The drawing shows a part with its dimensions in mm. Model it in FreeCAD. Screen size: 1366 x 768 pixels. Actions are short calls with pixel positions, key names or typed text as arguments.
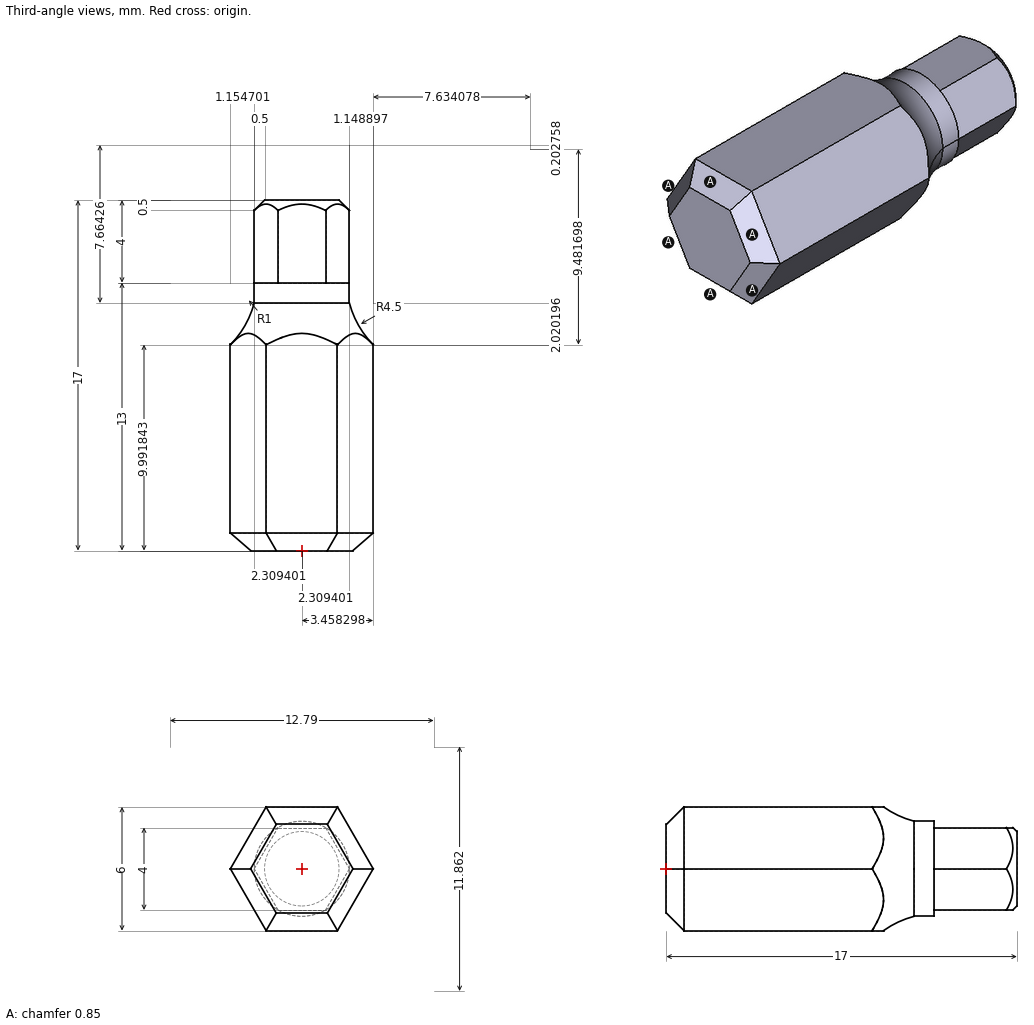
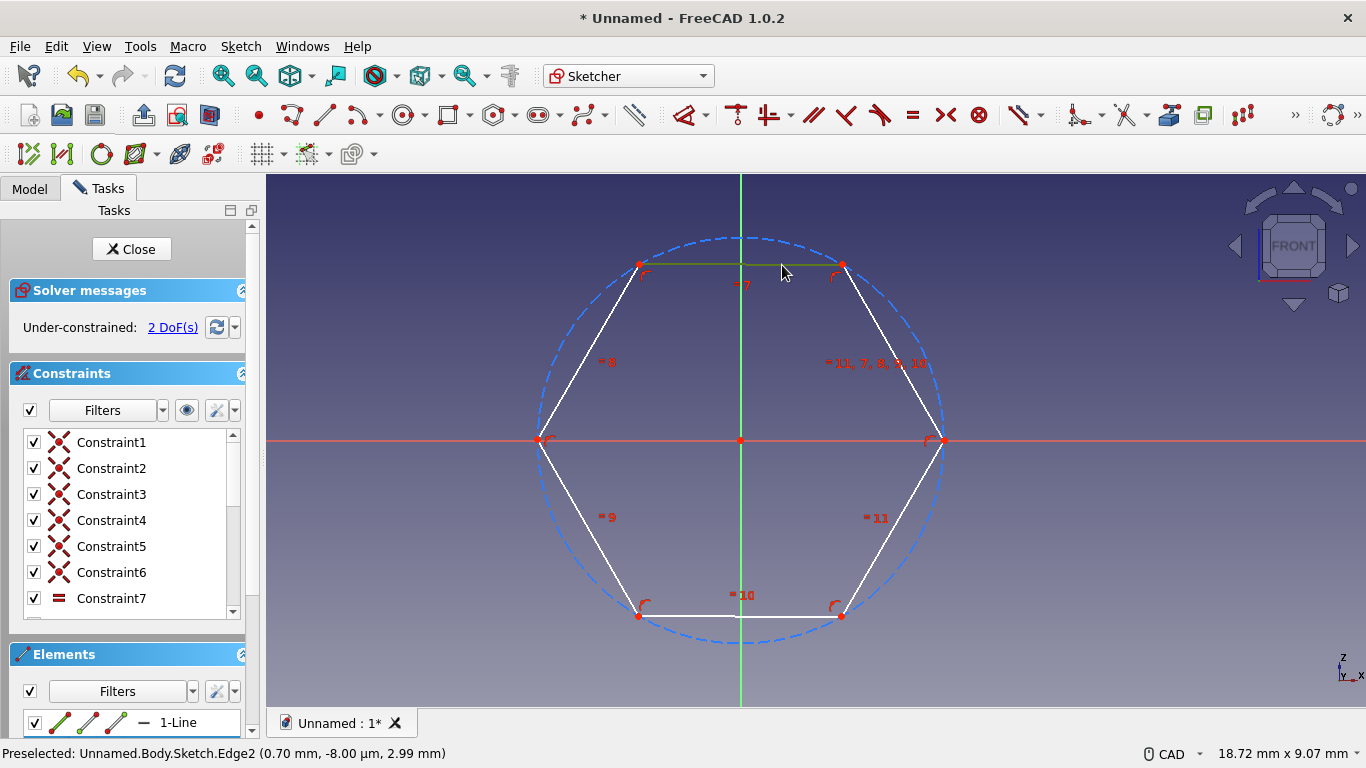
click(790, 116)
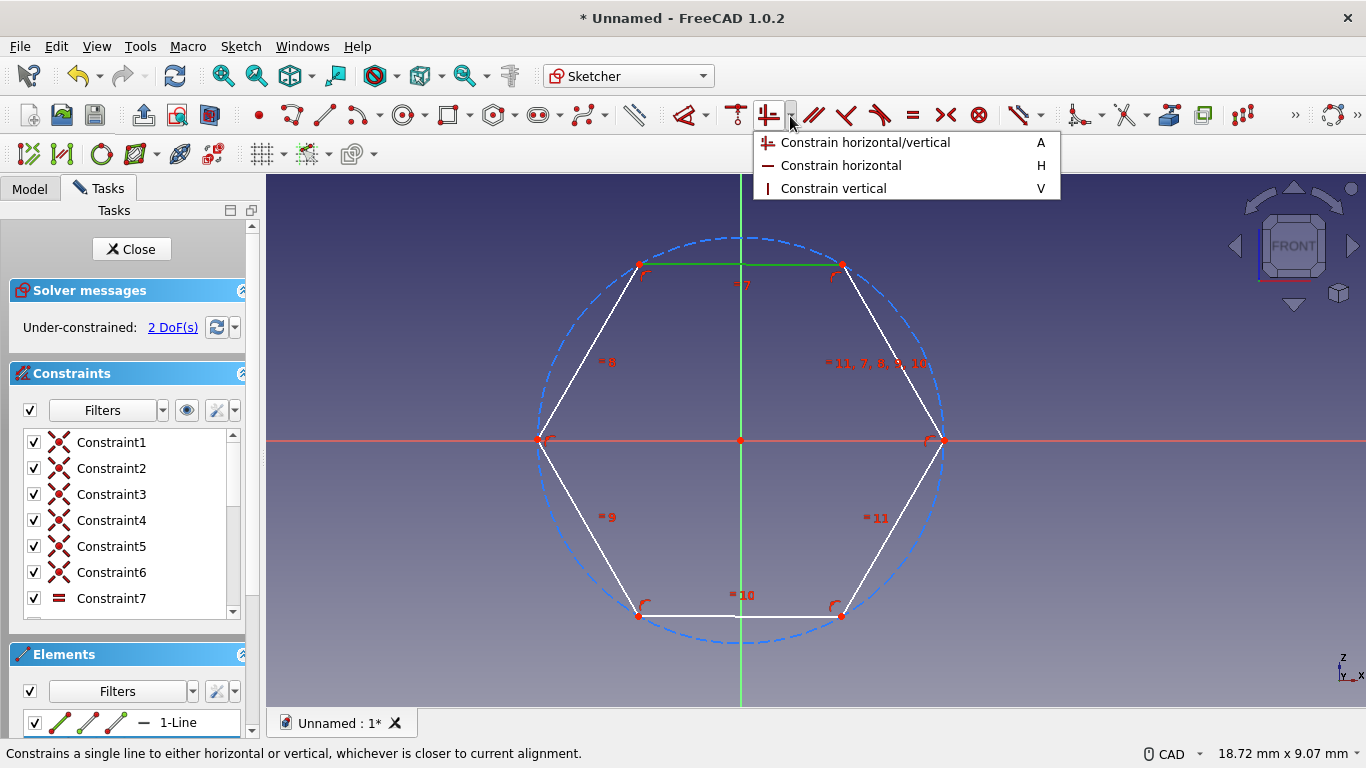
click(907, 166)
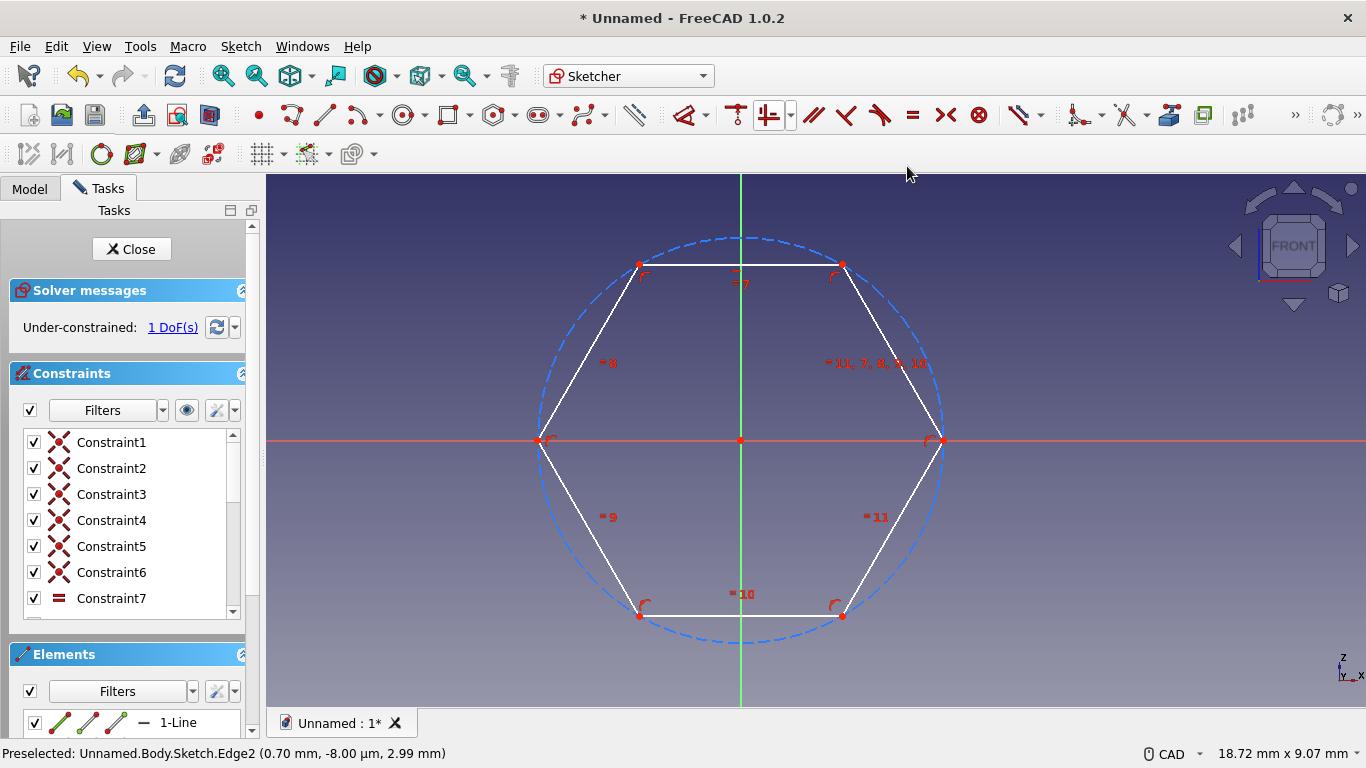
click(639, 616)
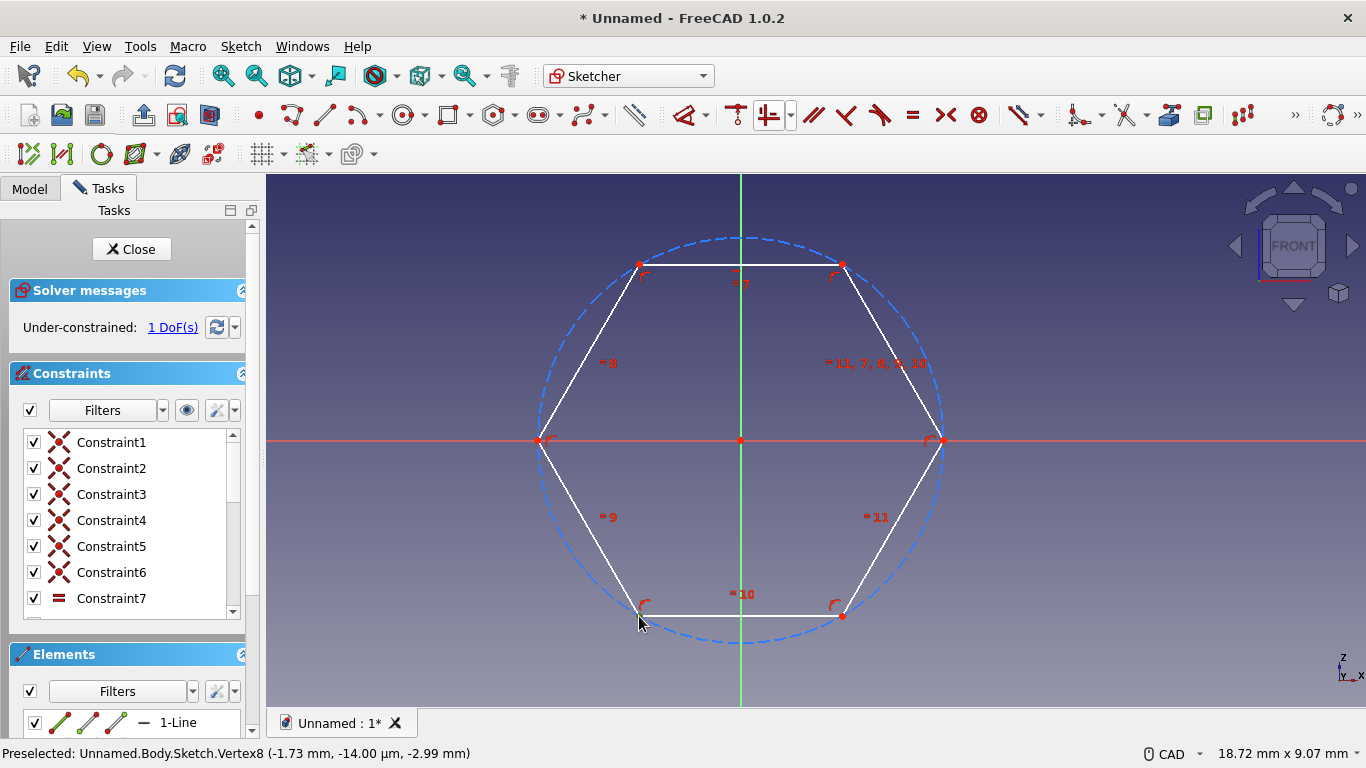
click(842, 265)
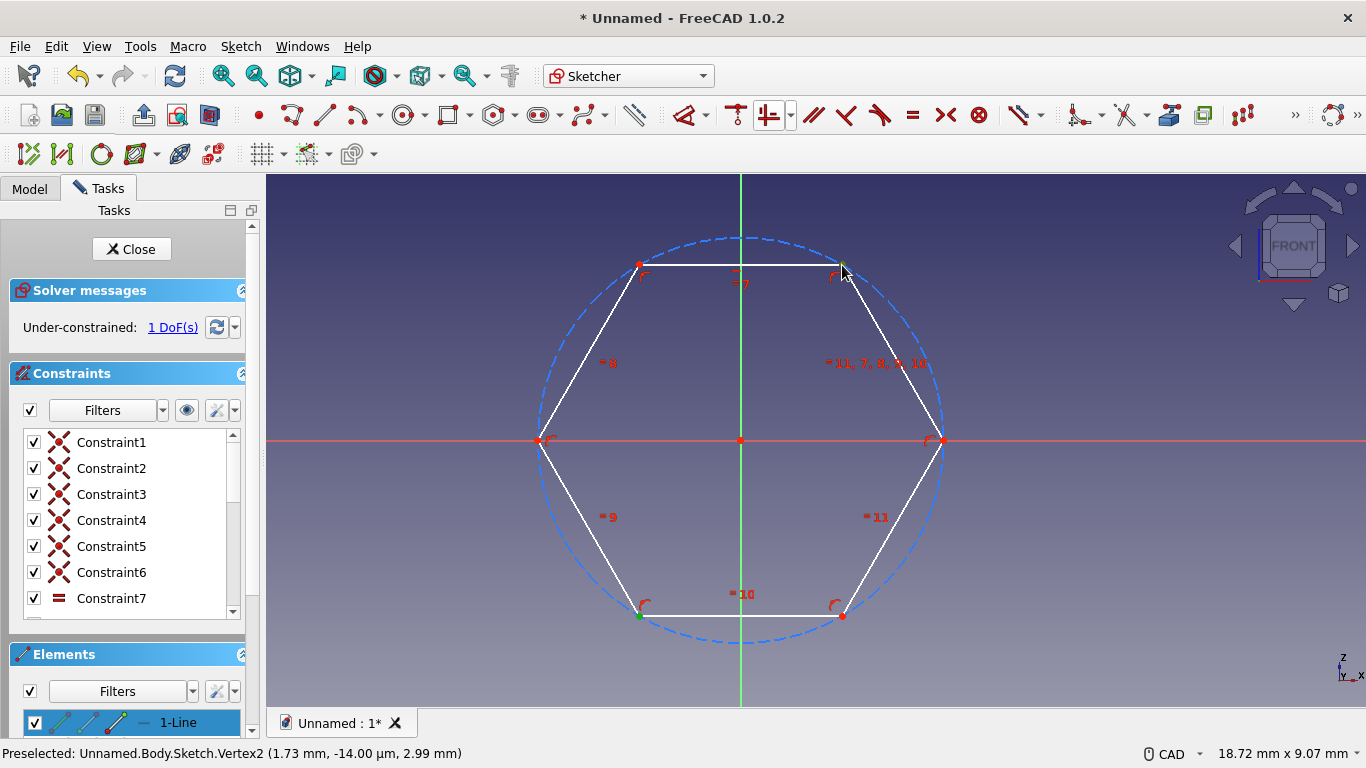
click(706, 116)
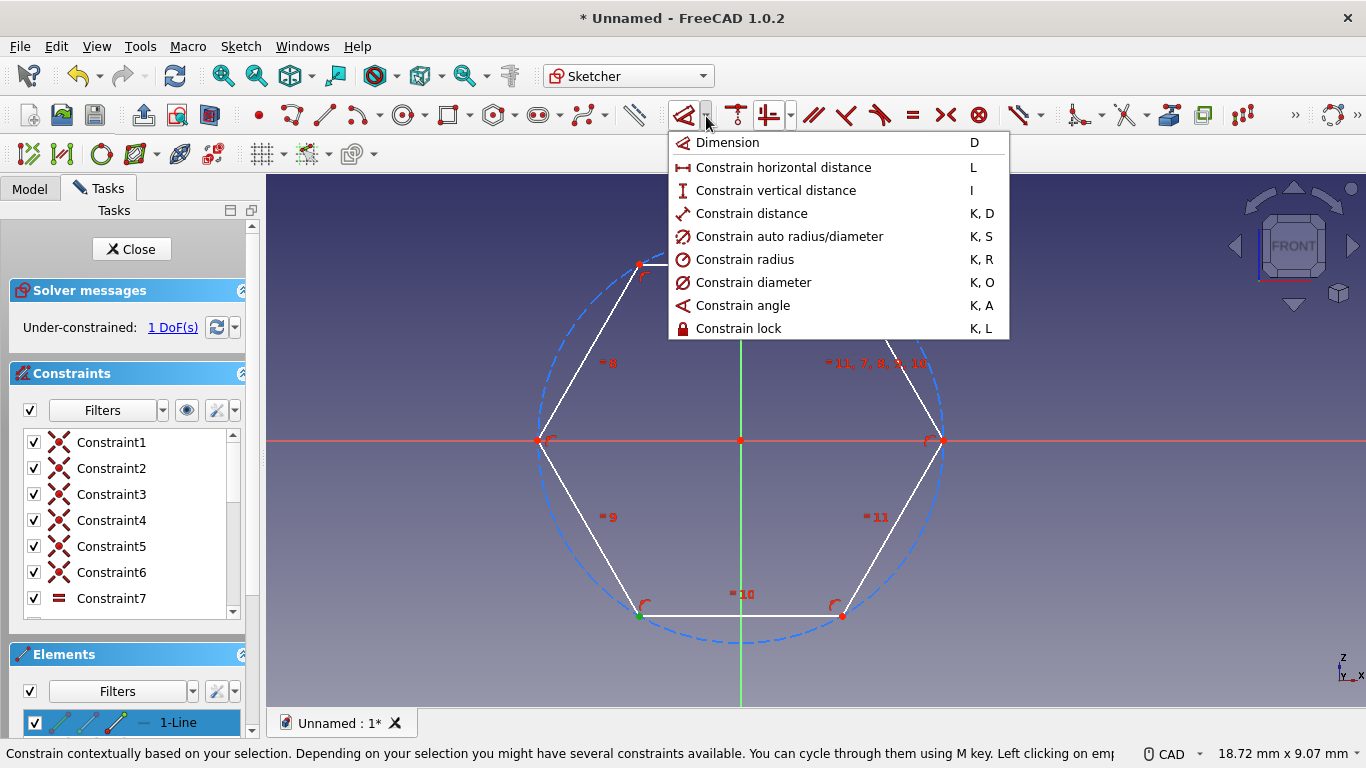
click(839, 190)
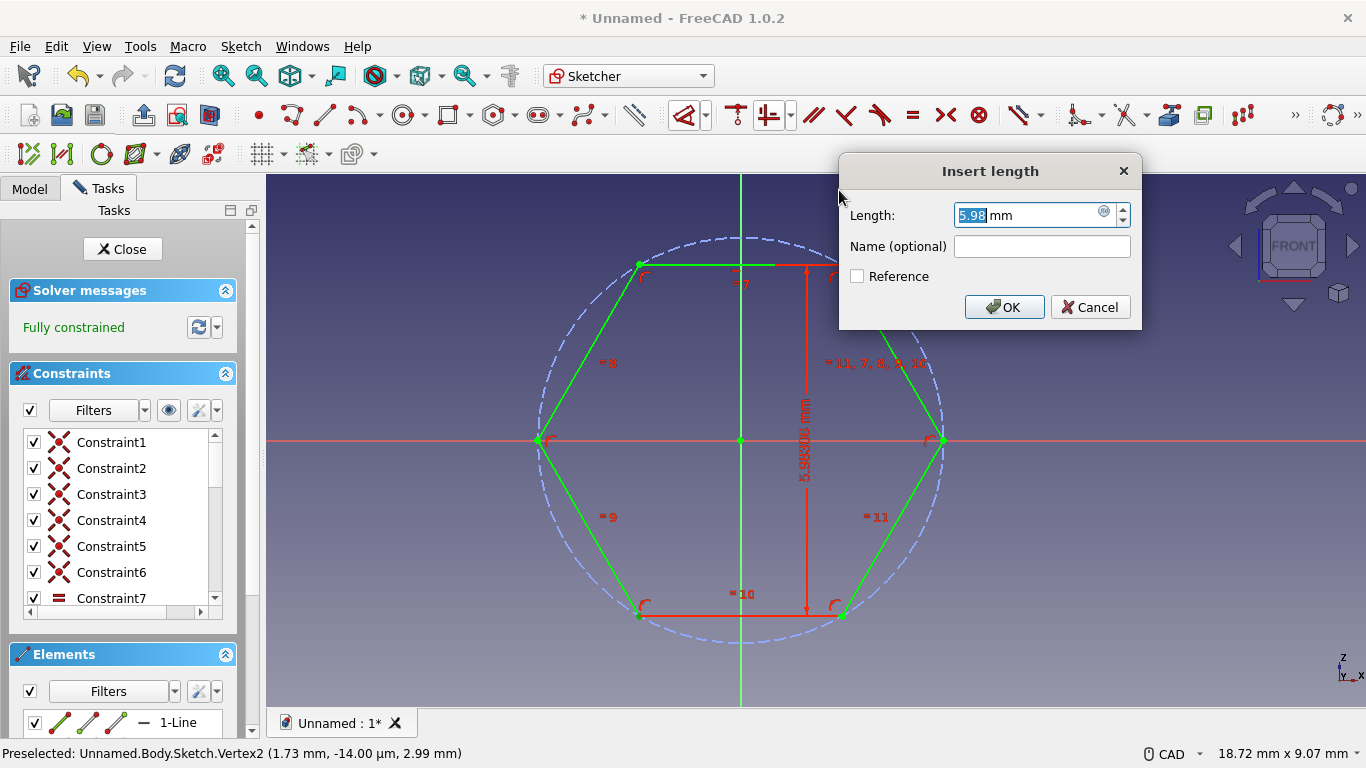
text(6)
key(Return)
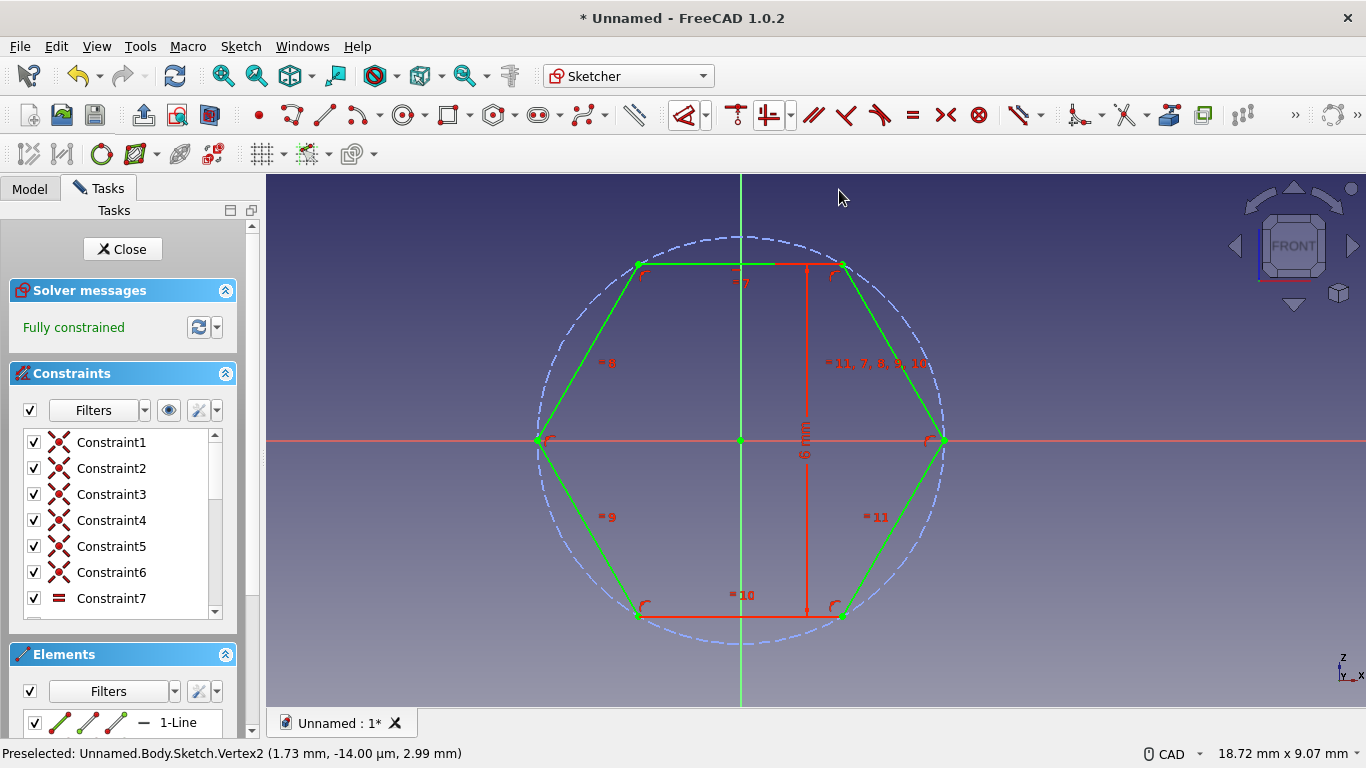
click(123, 249)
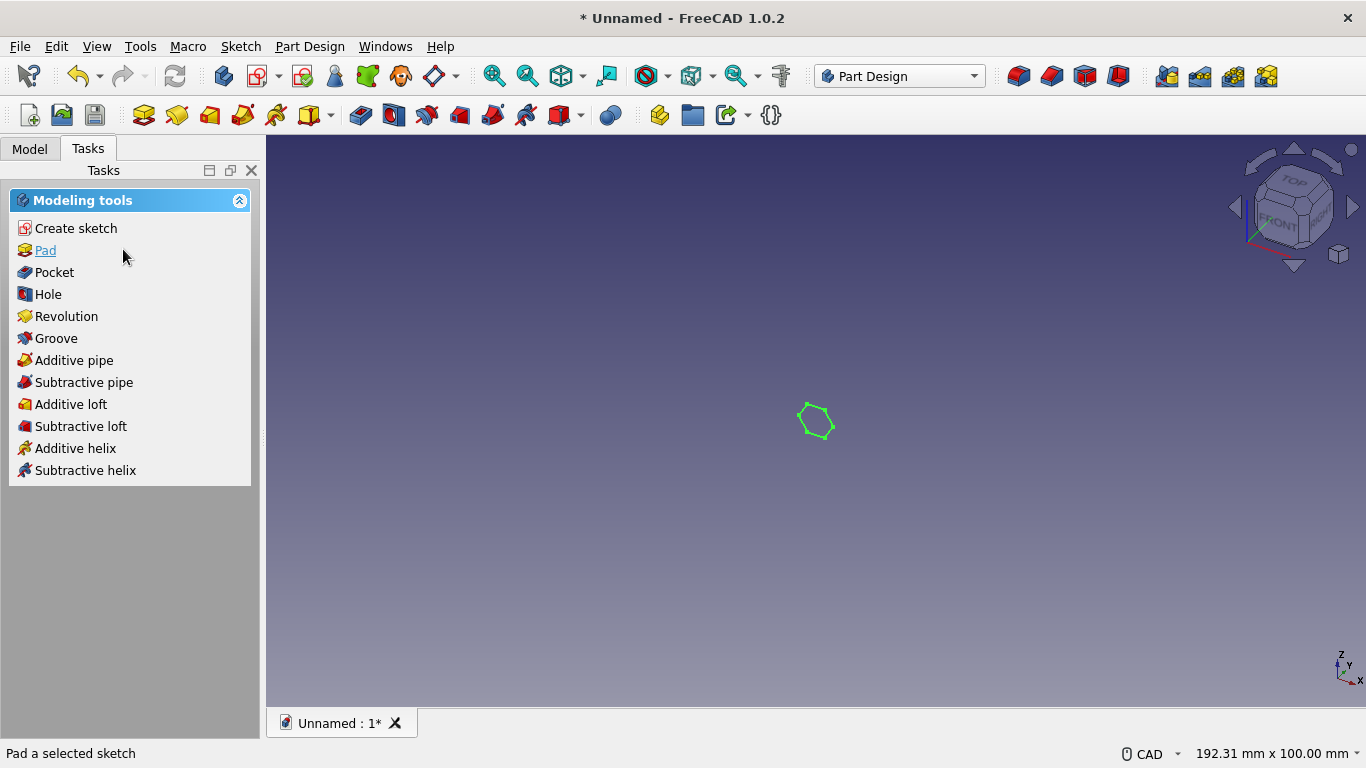
click(144, 116)